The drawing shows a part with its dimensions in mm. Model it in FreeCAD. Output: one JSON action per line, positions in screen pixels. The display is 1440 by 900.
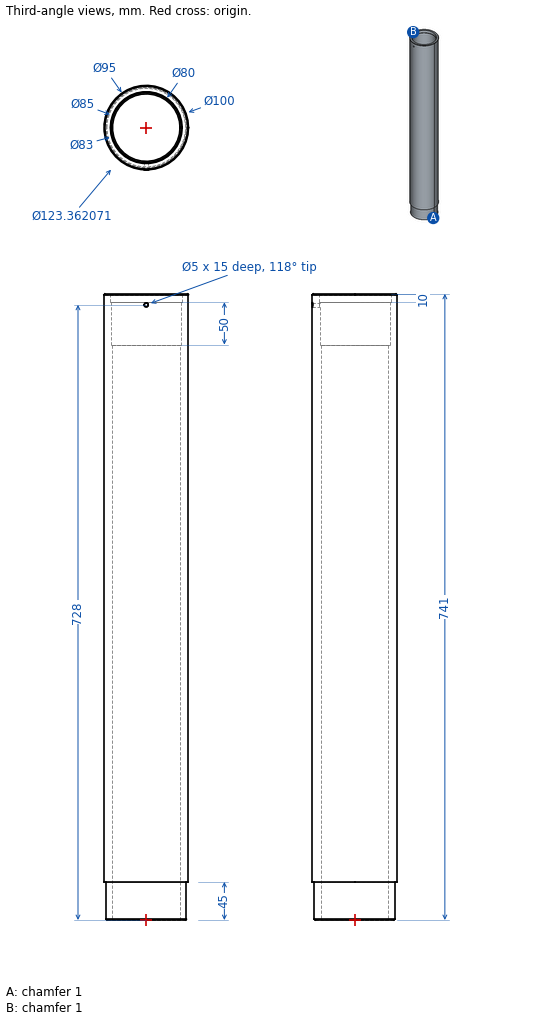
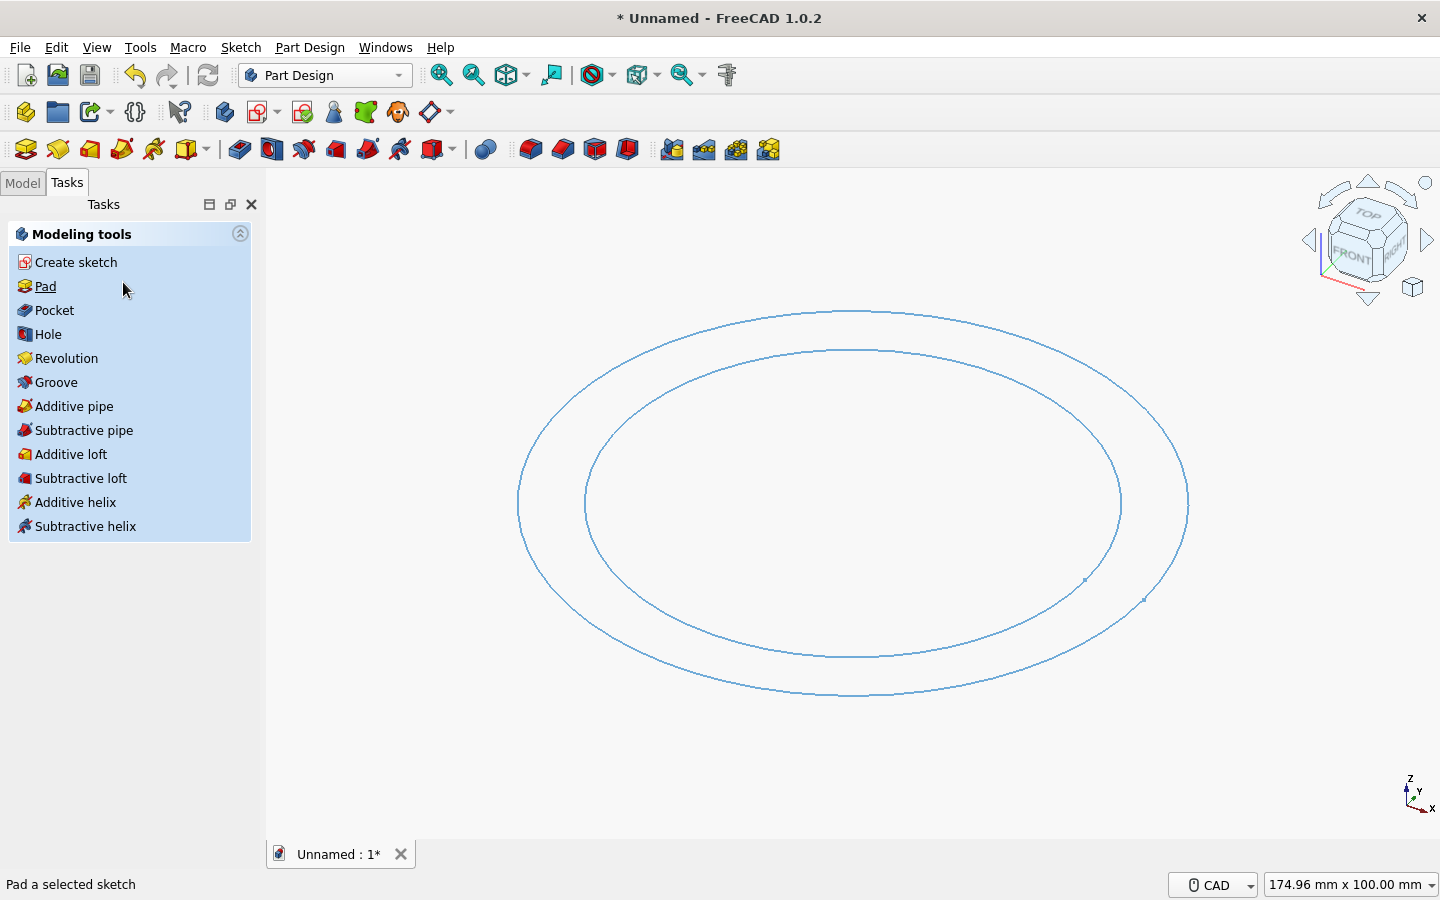
{"action": "left_click", "coordinate": [26, 150]}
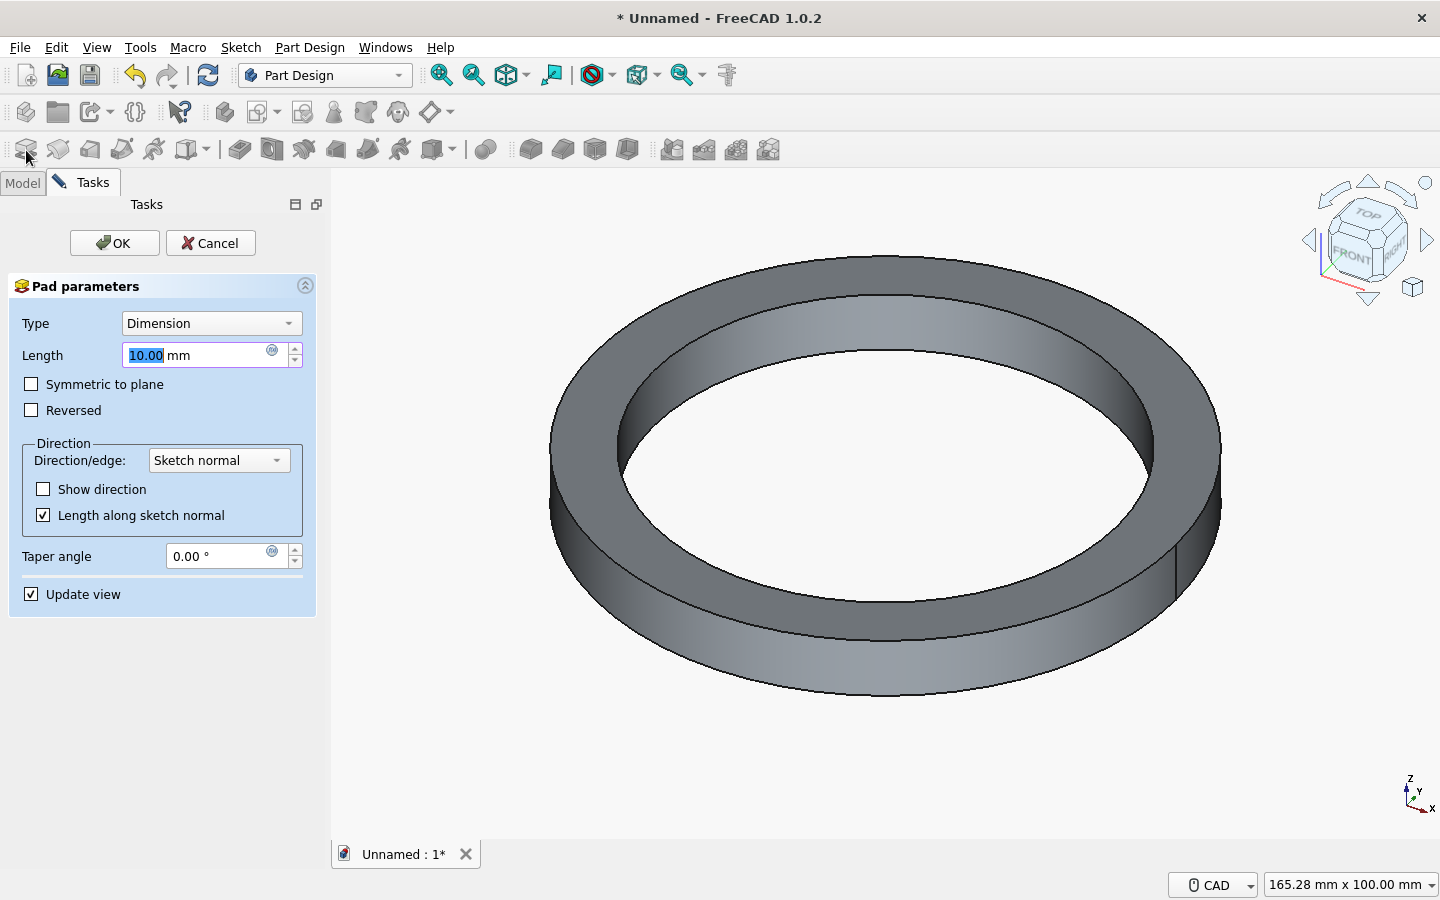
{"action": "type", "text": "741"}
{"action": "key", "text": "Tab"}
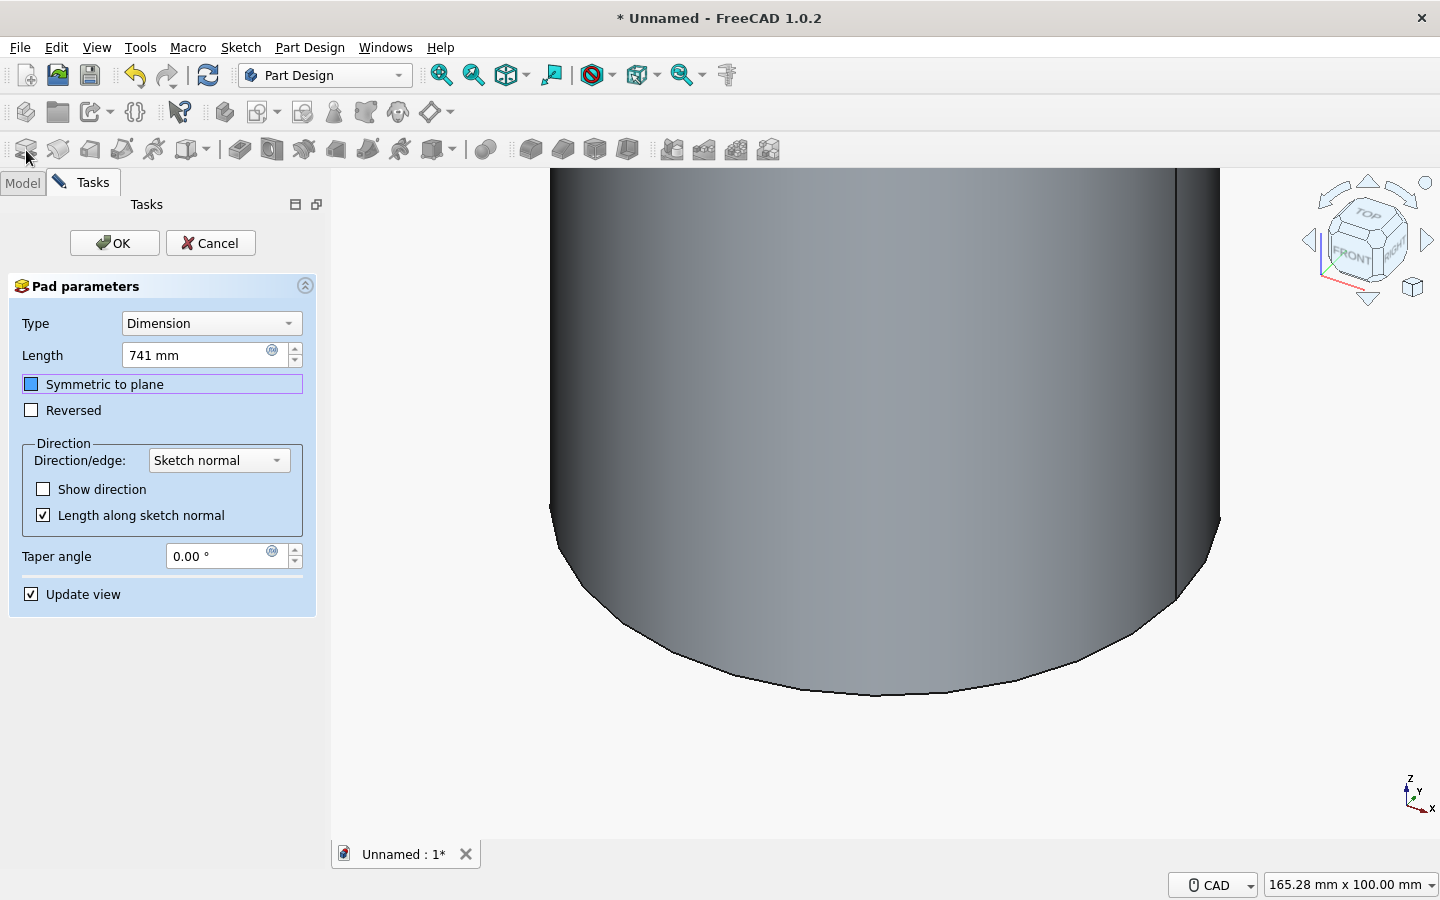
{"action": "left_click", "coordinate": [115, 243]}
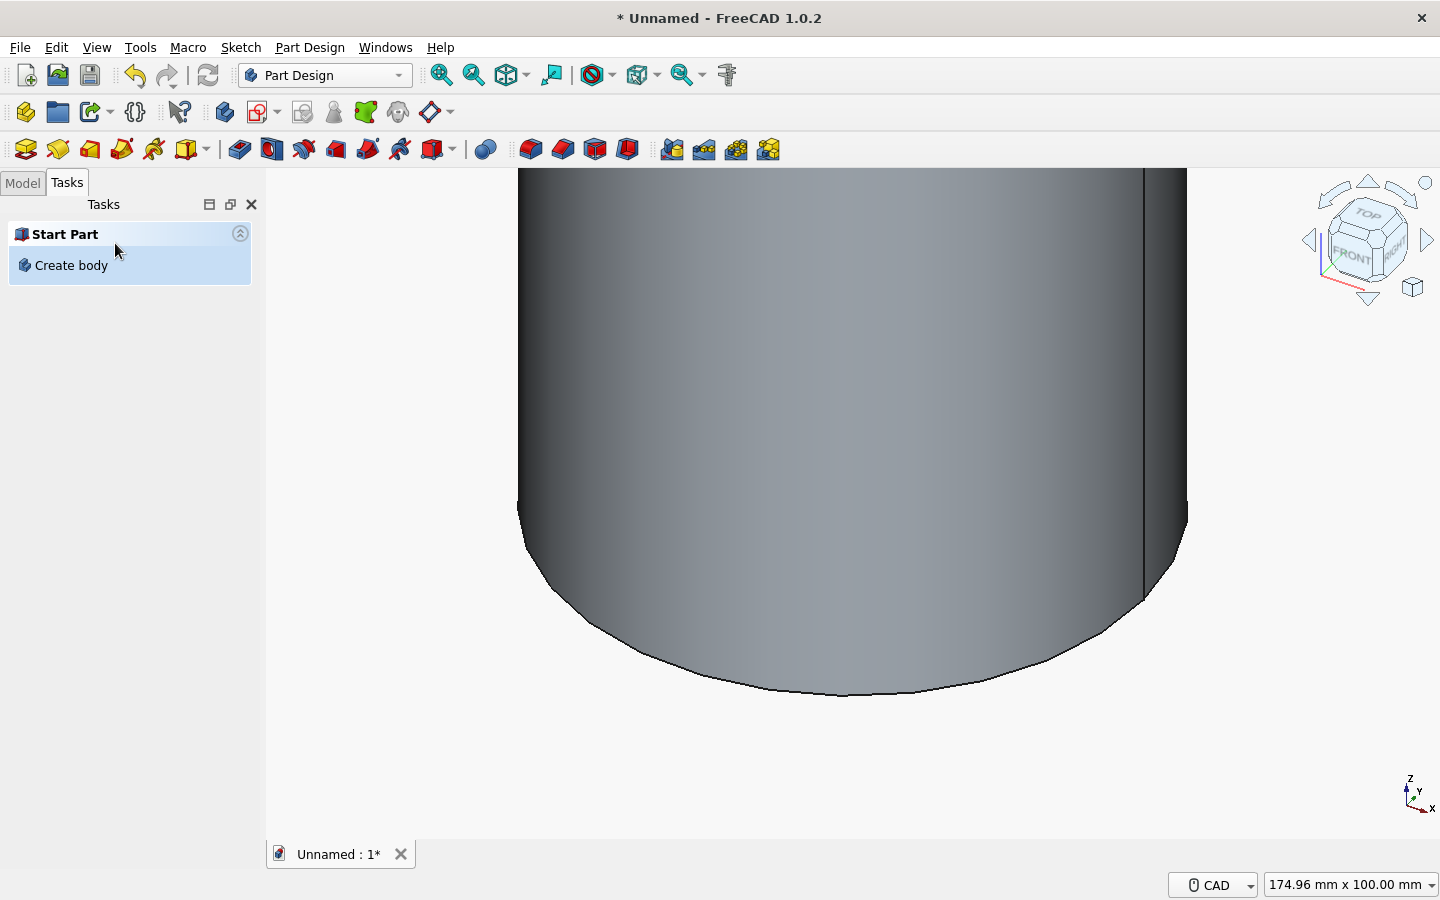
{"action": "left_click", "coordinate": [442, 76]}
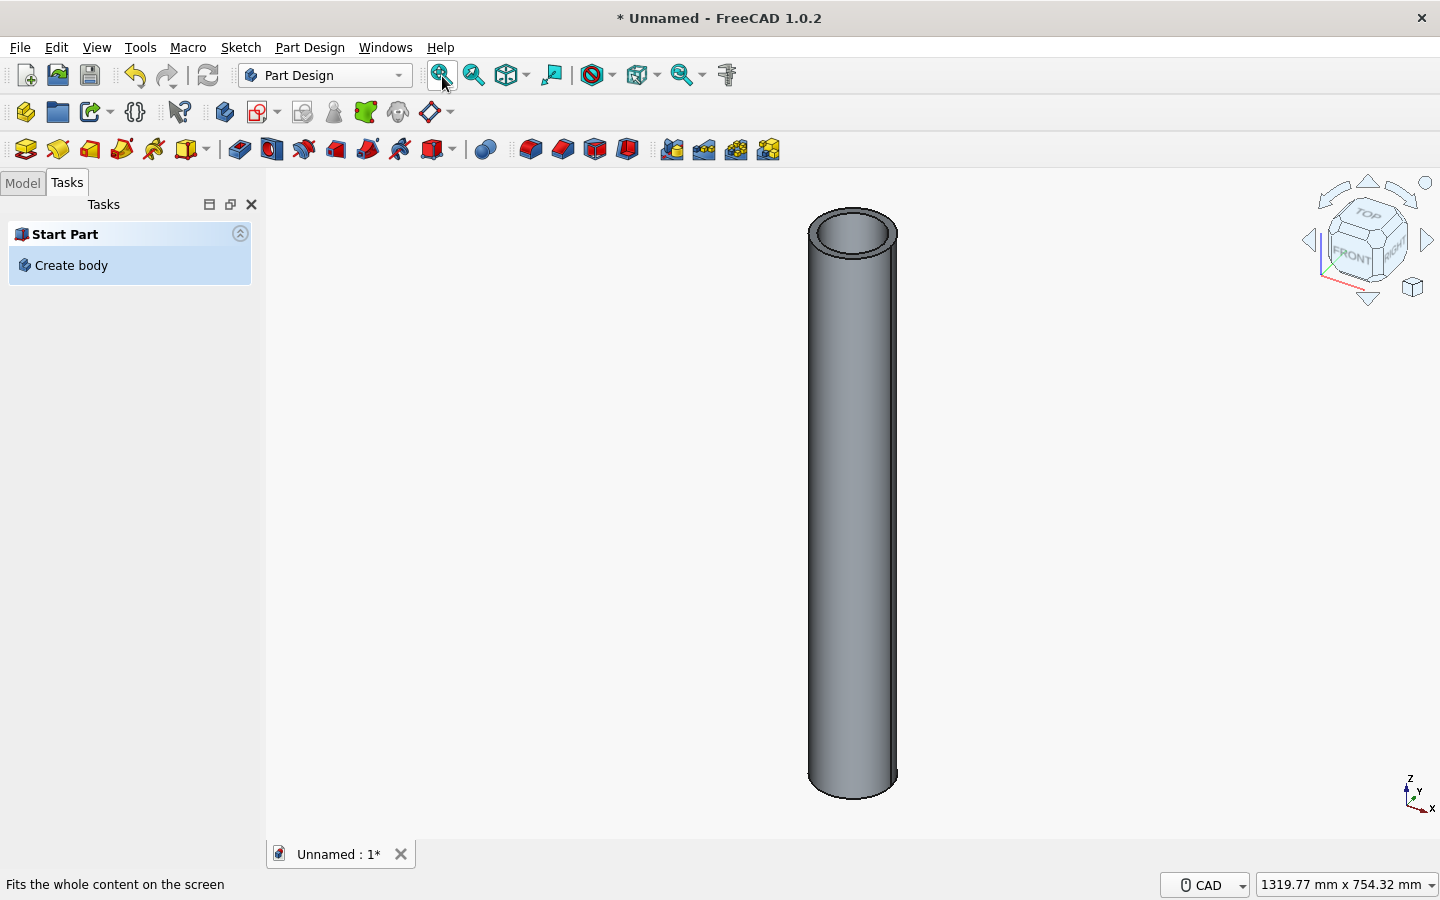
{"action": "key", "text": "5"}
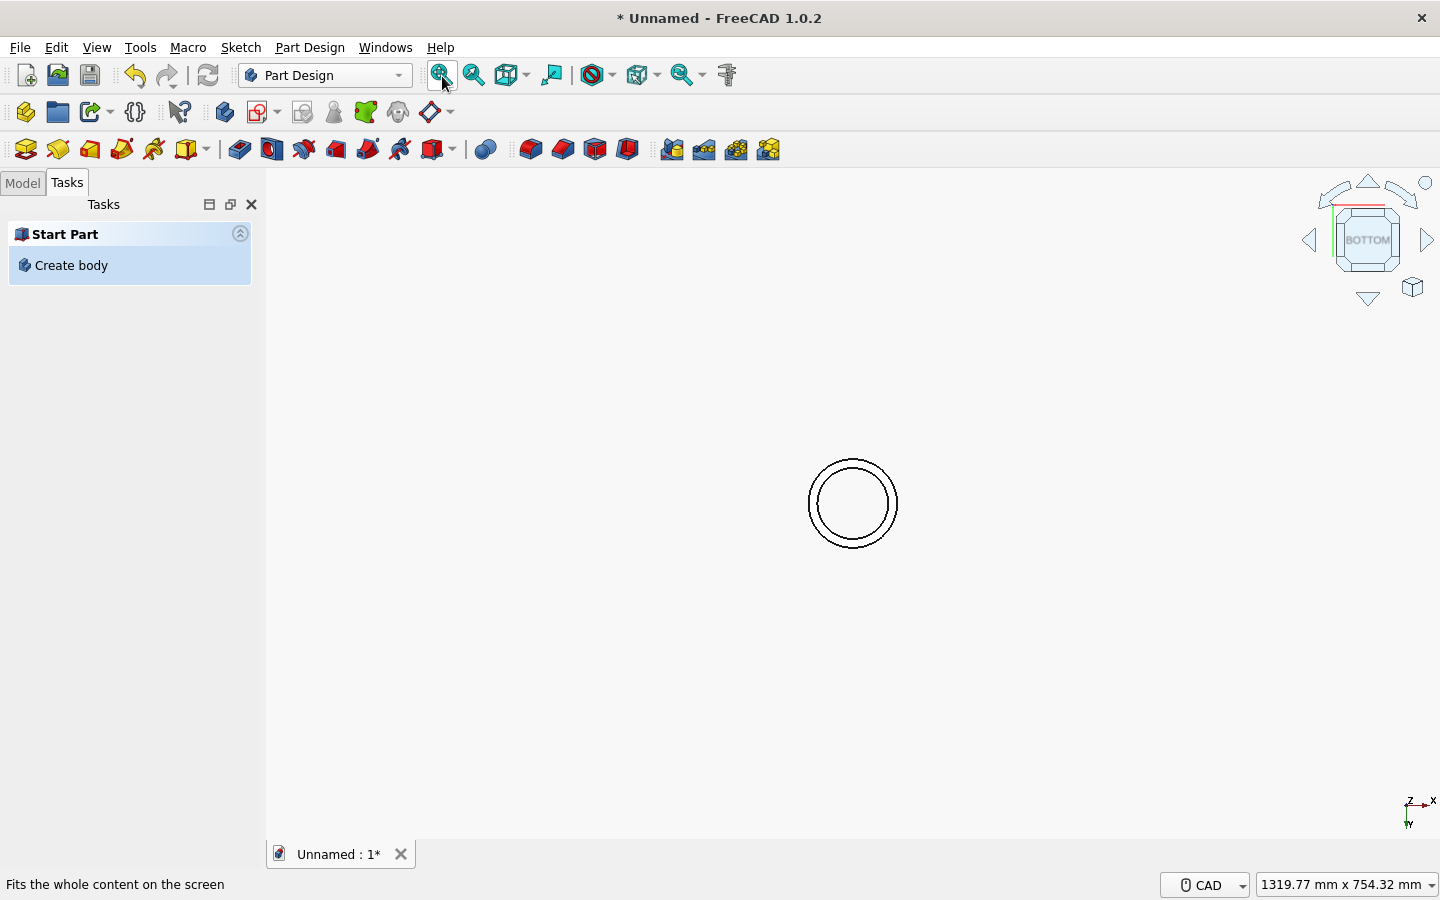
{"action": "left_click", "coordinate": [442, 76]}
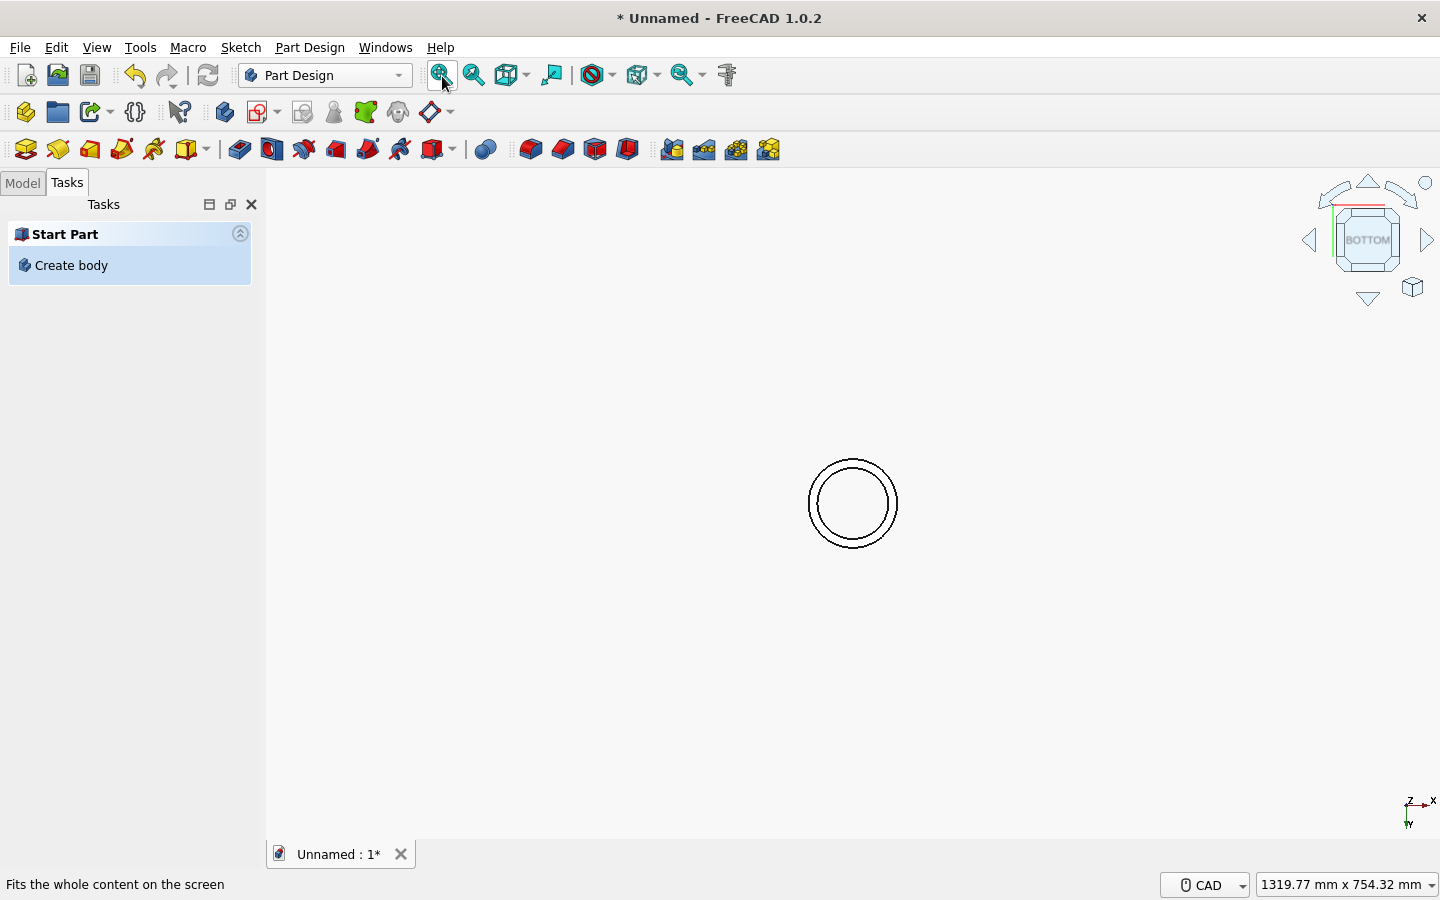
{"action": "scroll", "coordinate": [815, 490], "scroll_direction": "up", "scroll_amount": 6}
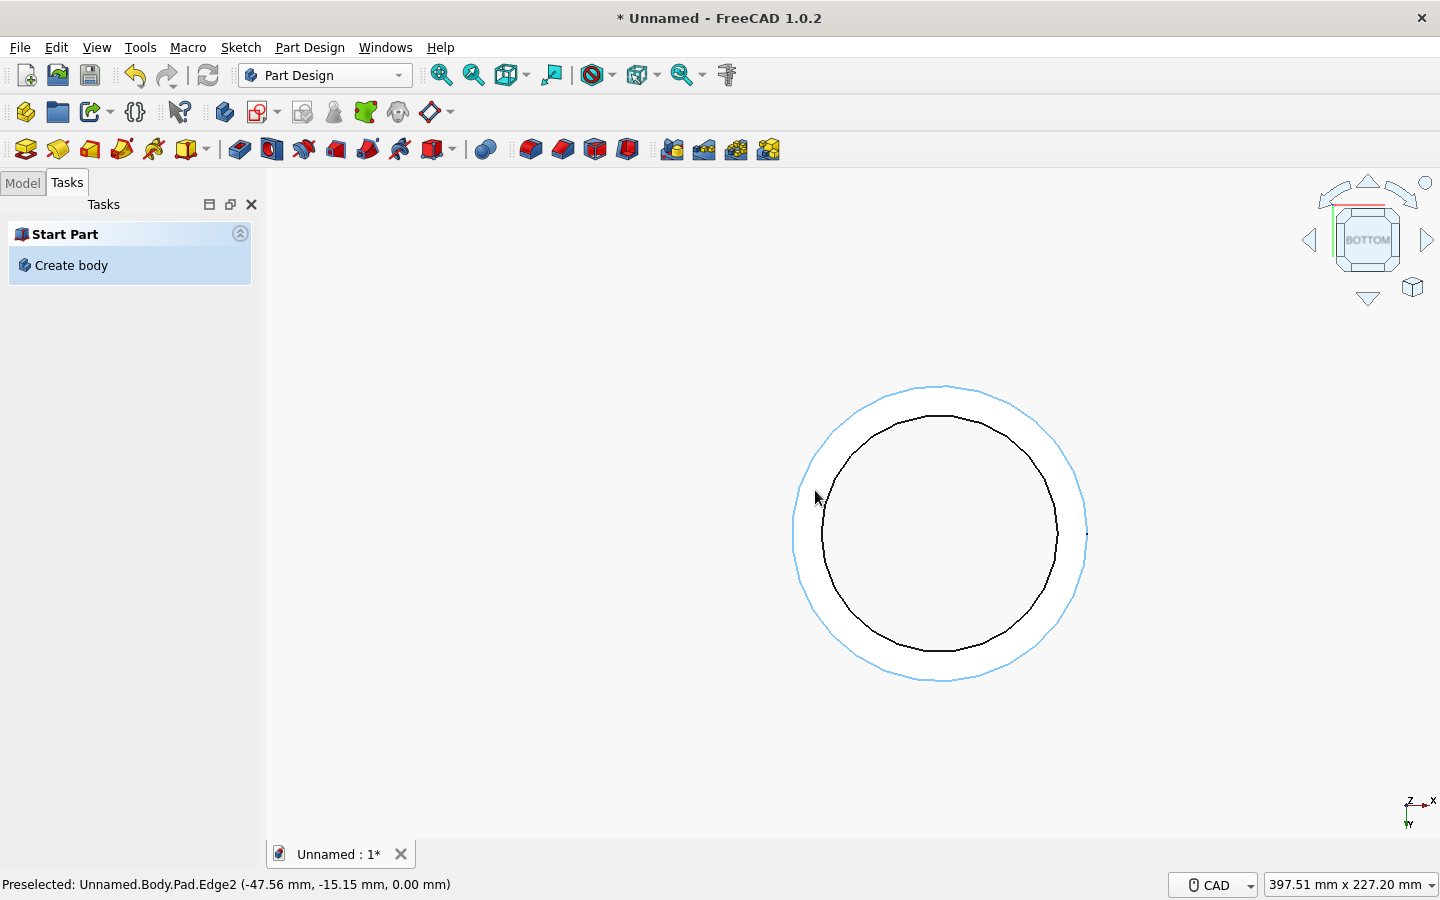
{"action": "left_click", "coordinate": [813, 491]}